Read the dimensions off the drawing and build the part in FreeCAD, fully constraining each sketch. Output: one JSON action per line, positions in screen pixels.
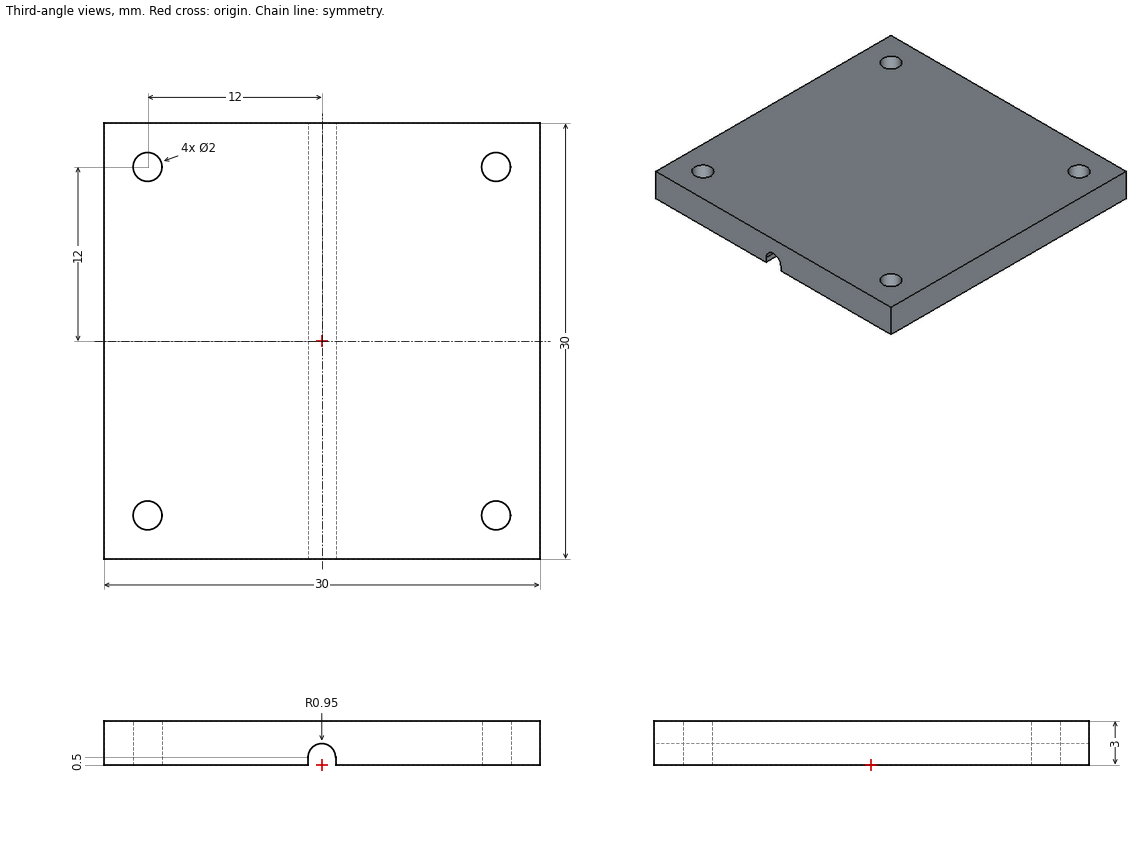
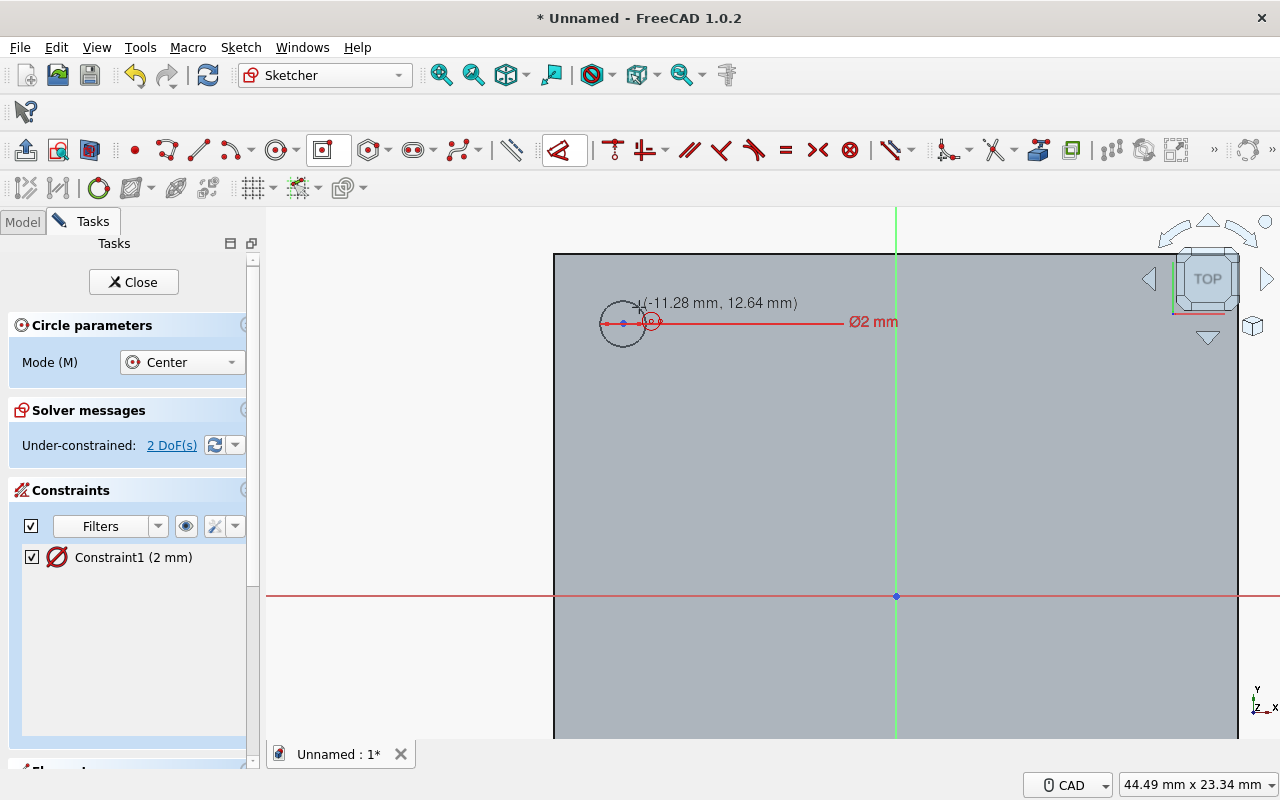
{"action": "scroll", "coordinate": [472, 323], "scroll_direction": "down", "scroll_amount": 3}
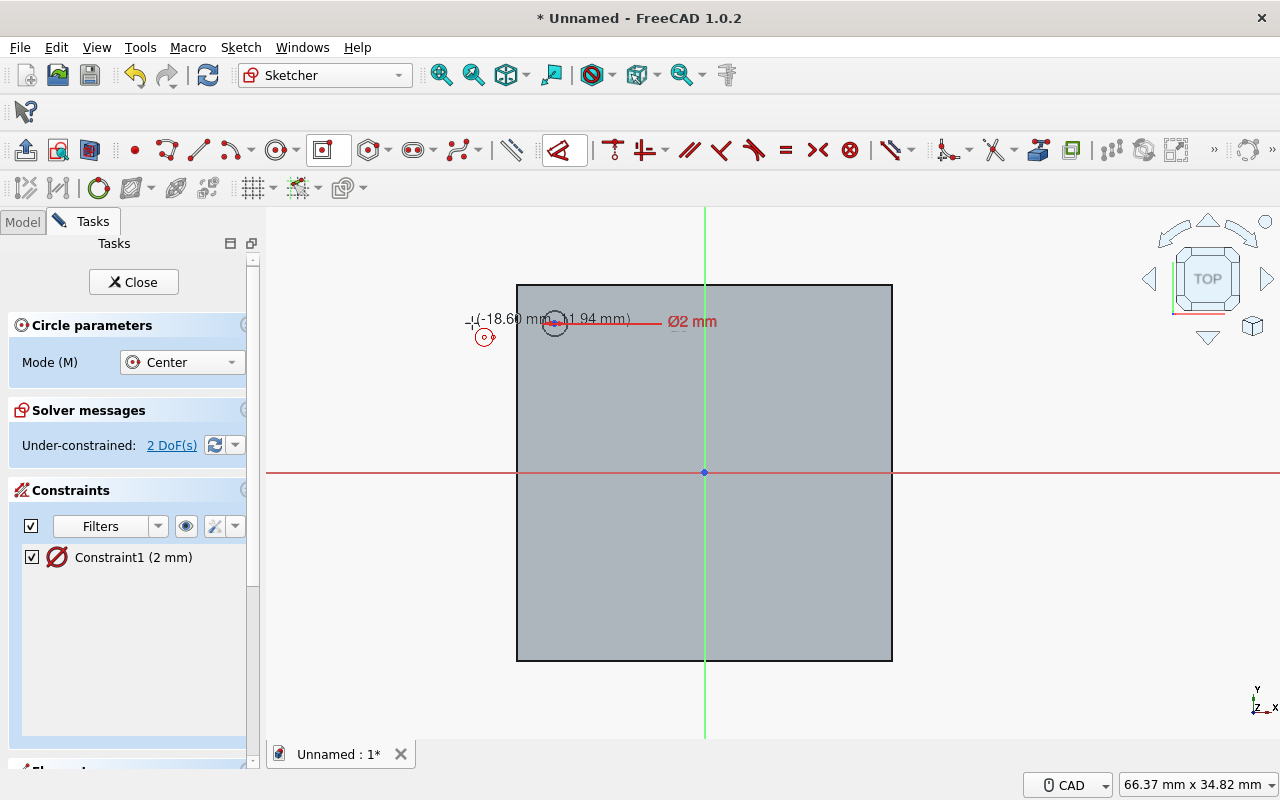
{"action": "scroll", "coordinate": [855, 323], "scroll_direction": "up", "scroll_amount": 3}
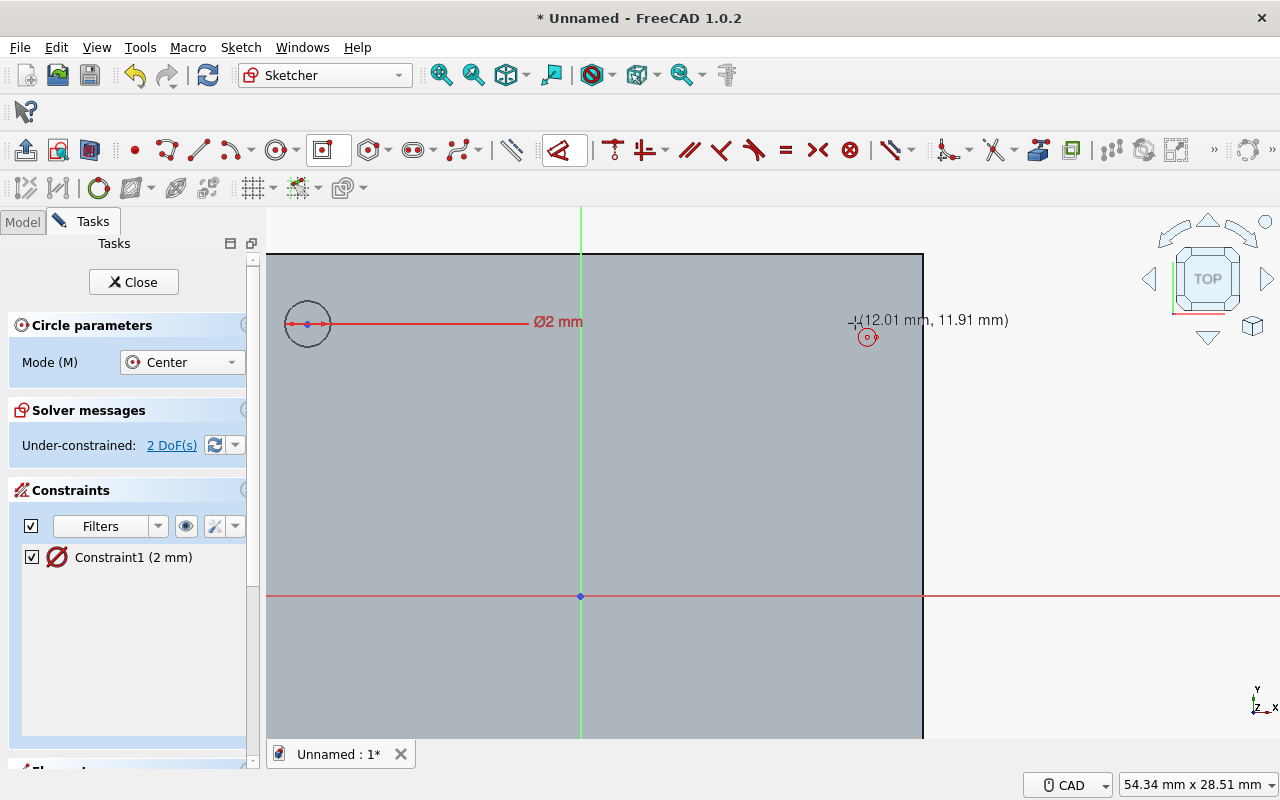
{"action": "left_click", "coordinate": [854, 323]}
{"action": "mouse_move", "coordinate": [870, 307]}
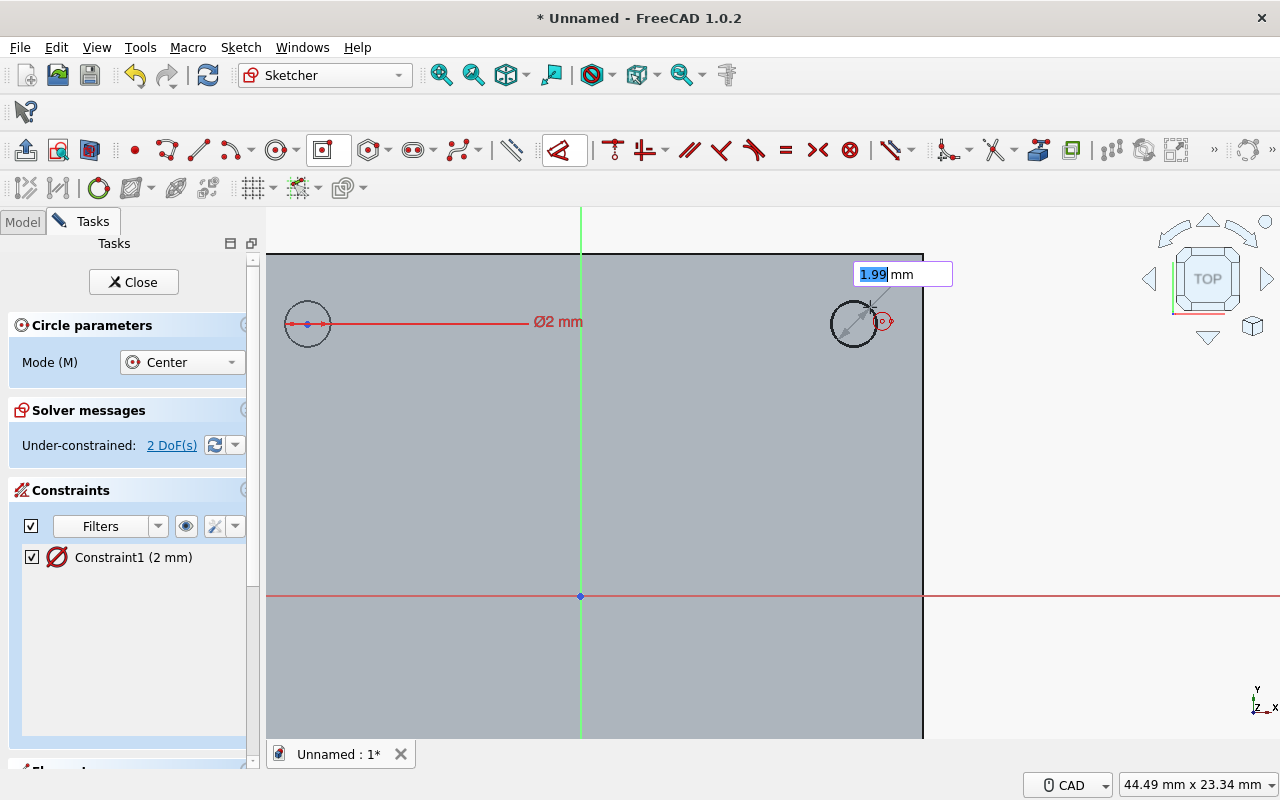
{"action": "type", "text": "2"}
{"action": "key", "text": "Return"}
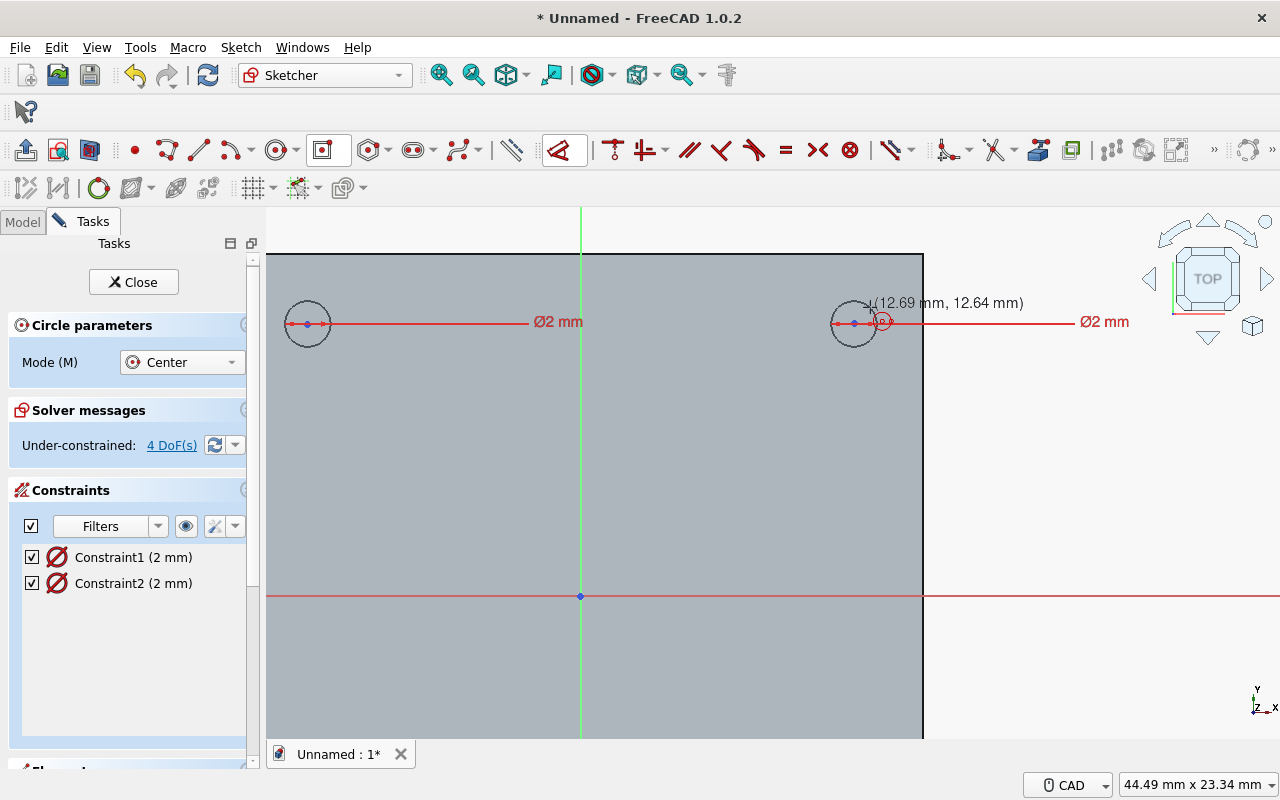
{"action": "scroll", "coordinate": [855, 323], "scroll_direction": "down", "scroll_amount": 3}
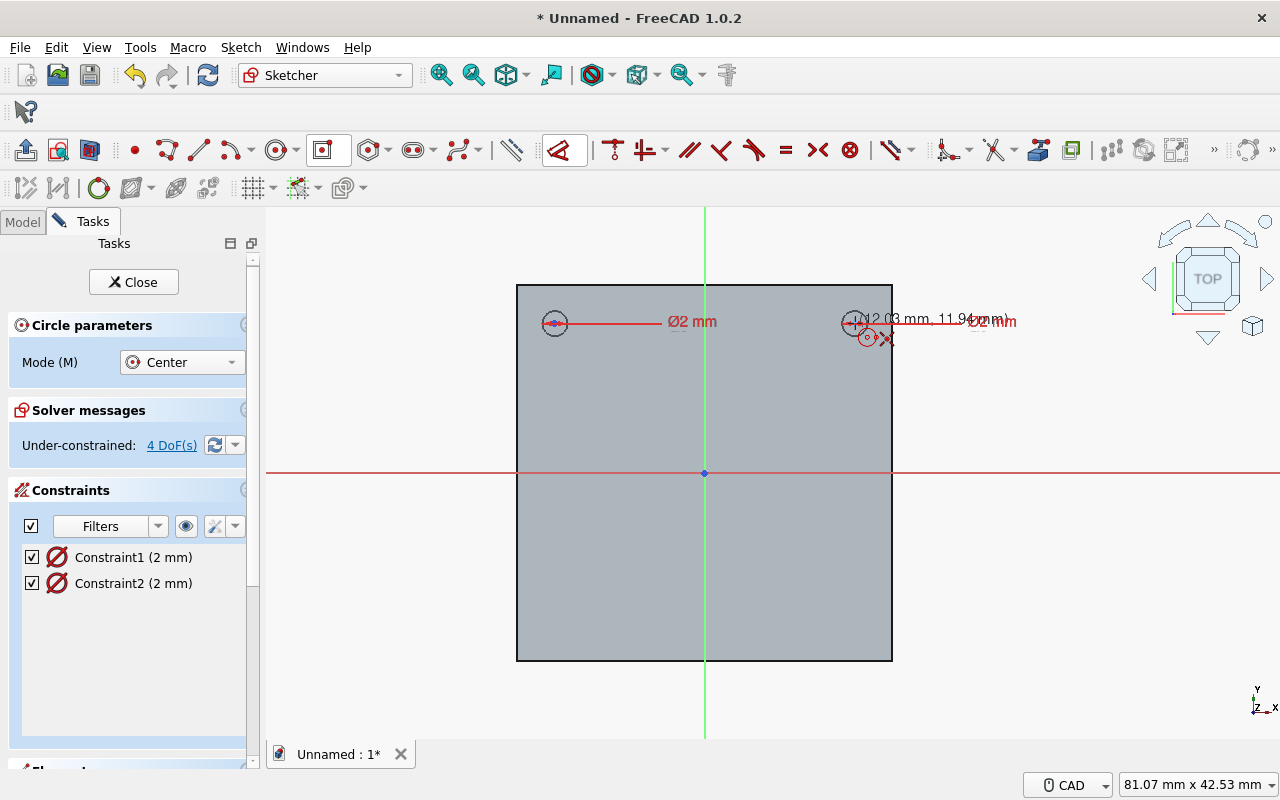
{"action": "scroll", "coordinate": [855, 623], "scroll_direction": "up", "scroll_amount": 3}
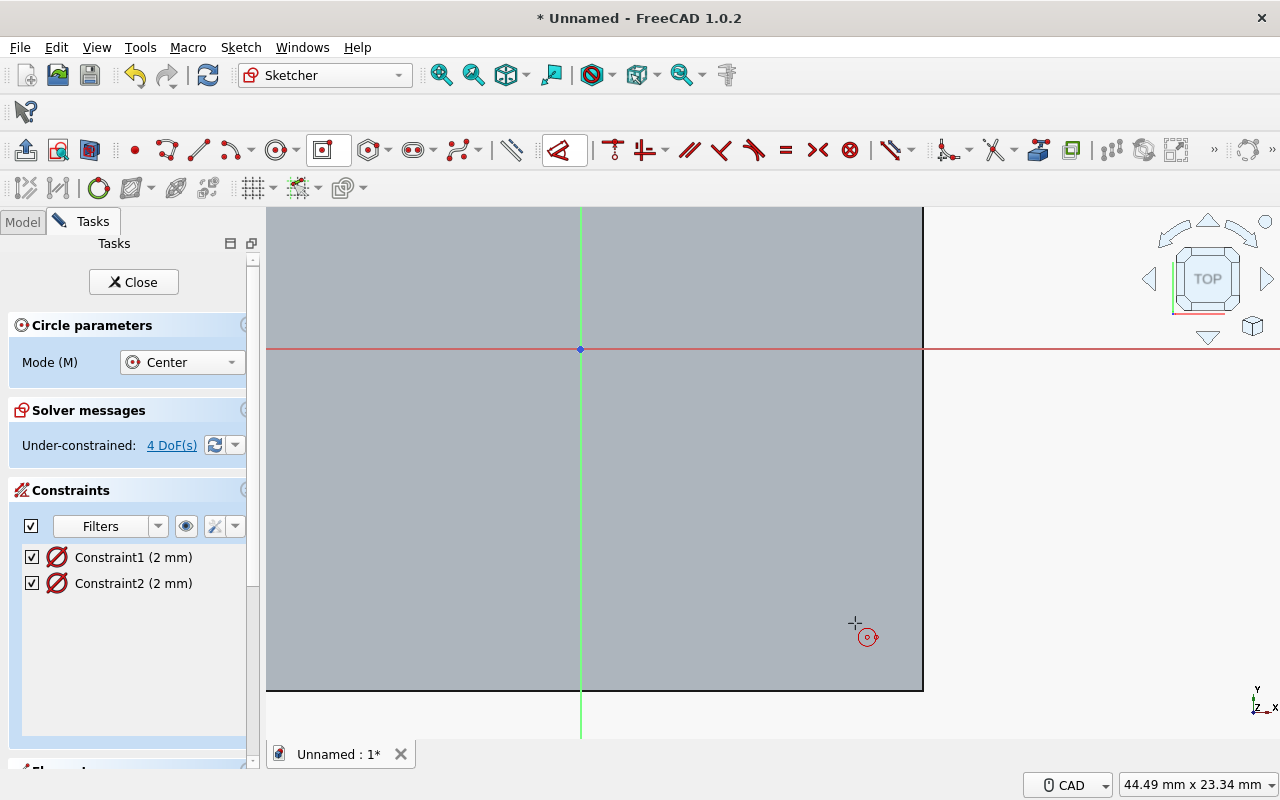
{"action": "left_click", "coordinate": [854, 623]}
{"action": "mouse_move", "coordinate": [870, 606]}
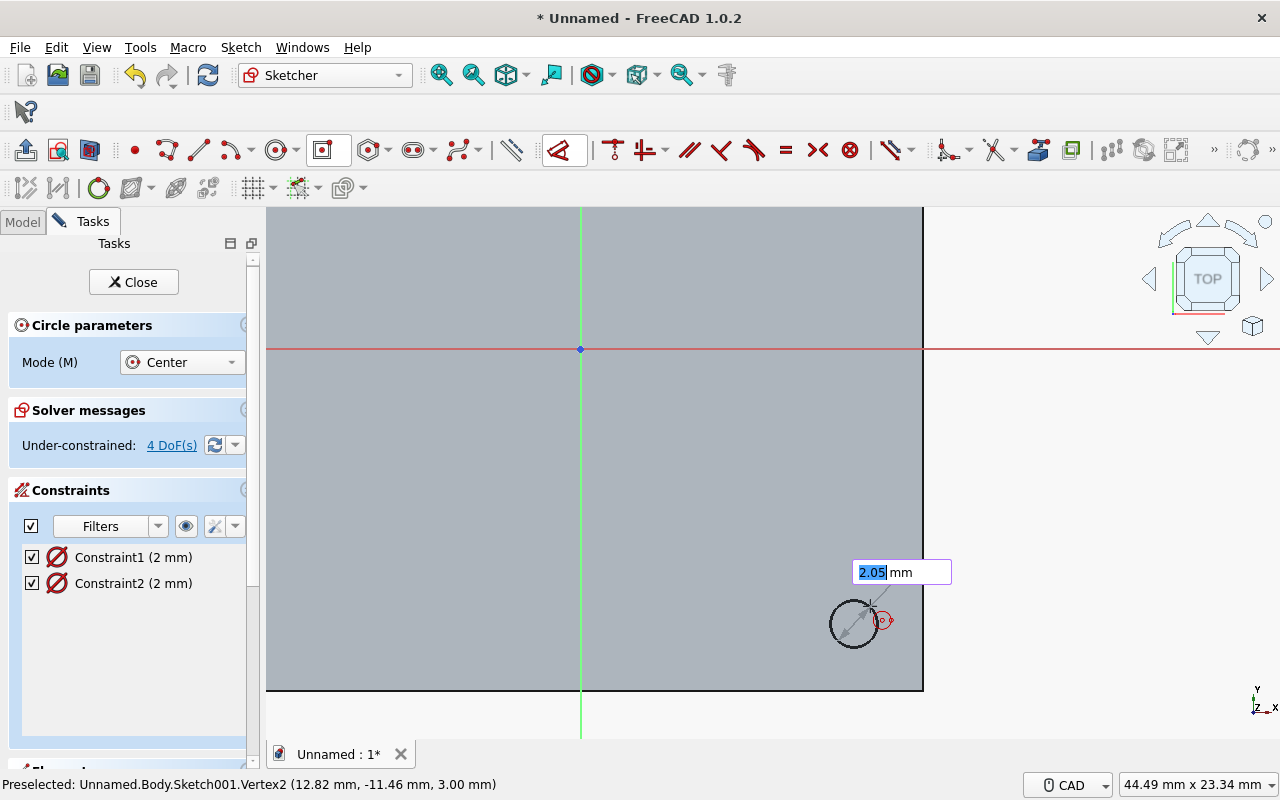
{"action": "type", "text": "2"}
{"action": "key", "text": "Return"}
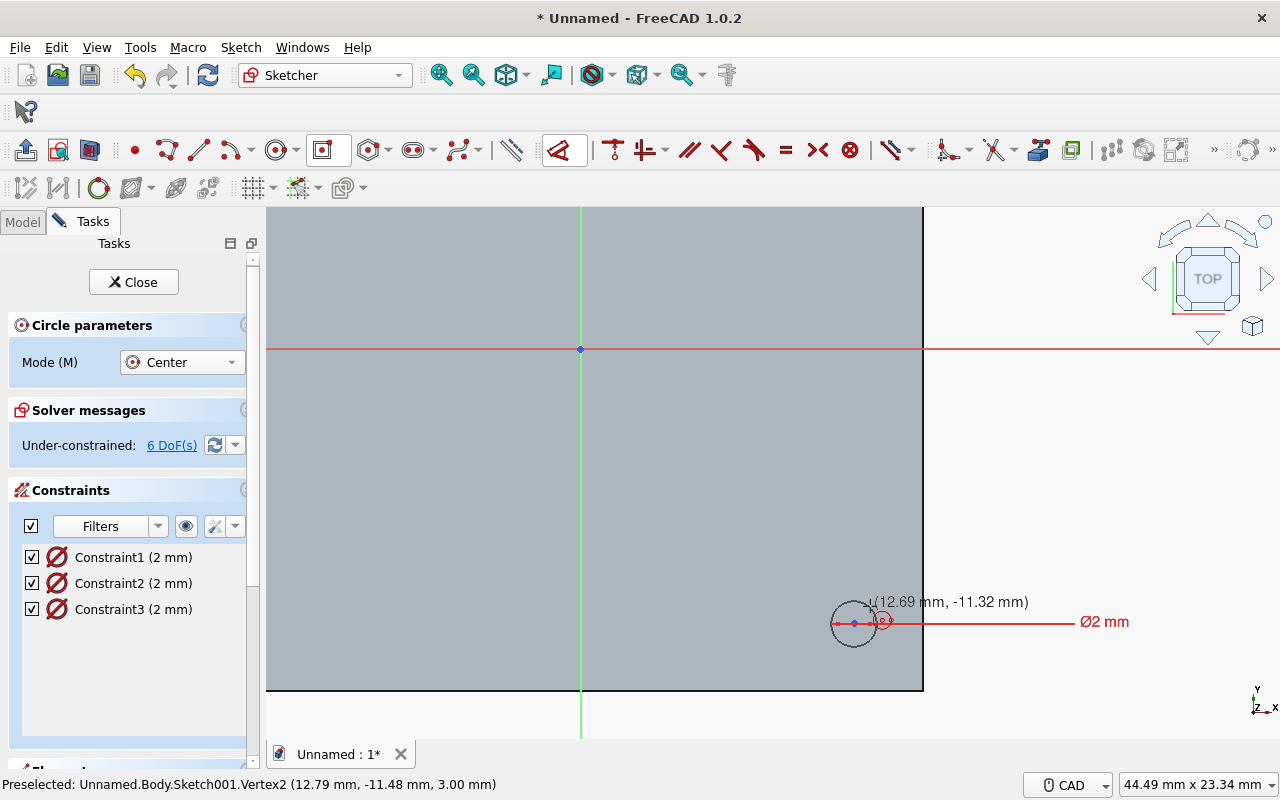
{"action": "left_click", "coordinate": [307, 623]}
{"action": "mouse_move", "coordinate": [323, 606]}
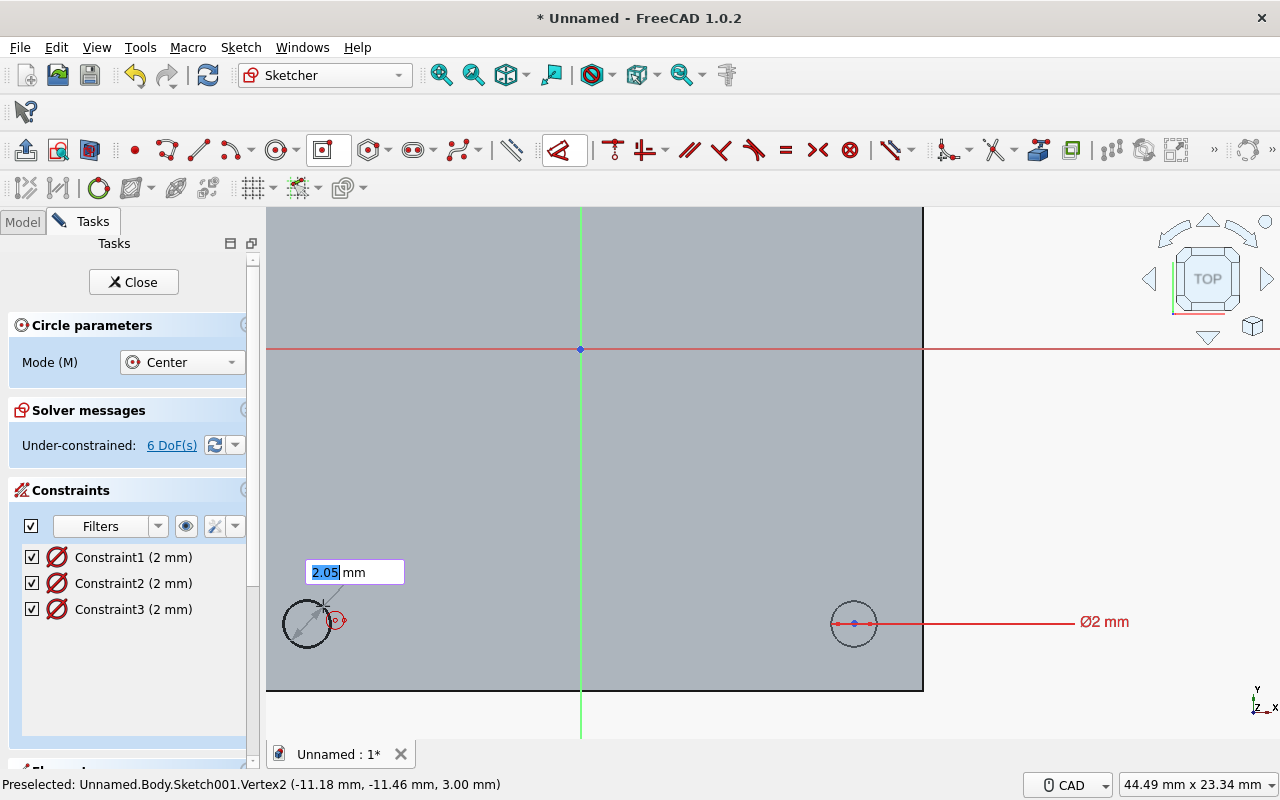
{"action": "type", "text": "2"}
{"action": "key", "text": "Return"}
{"action": "key", "text": "Escape"}